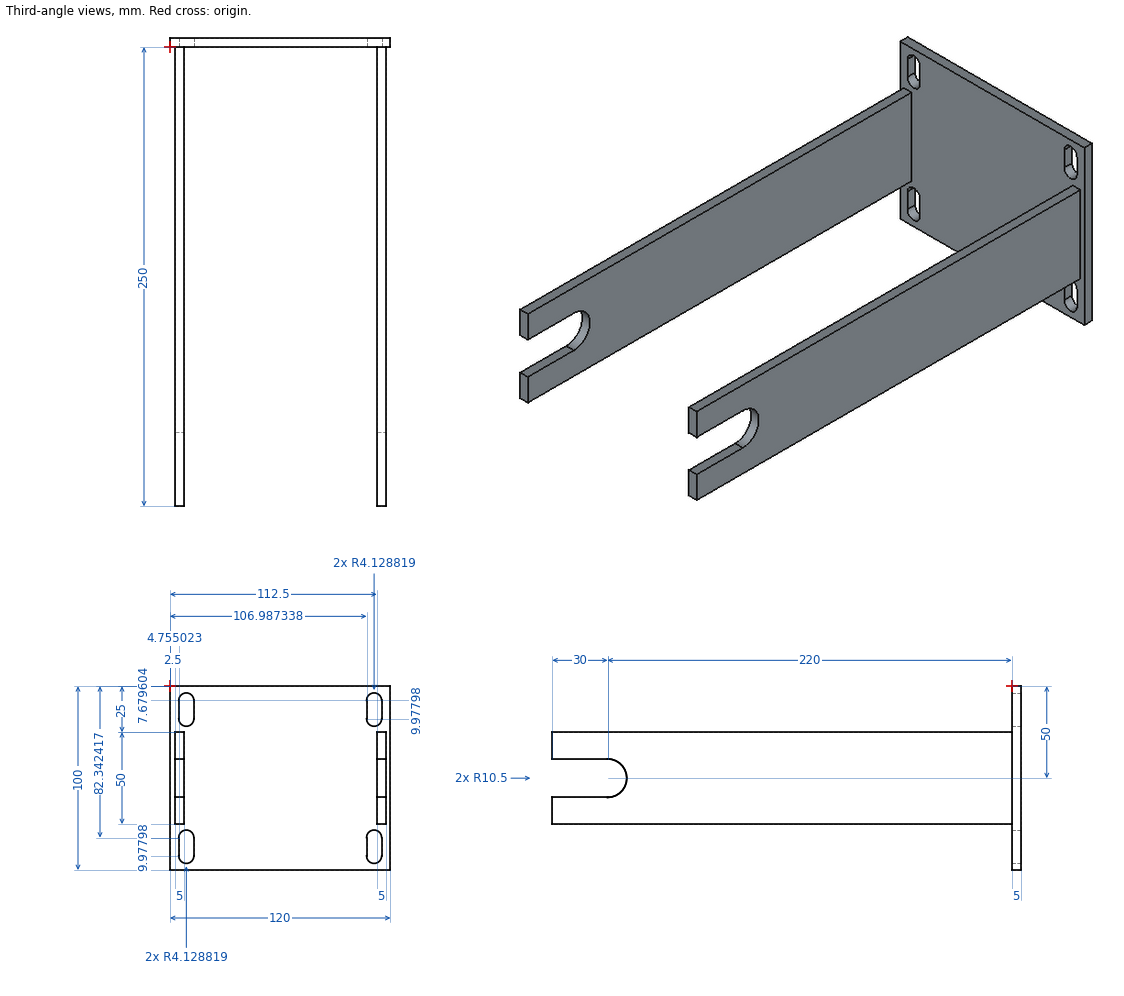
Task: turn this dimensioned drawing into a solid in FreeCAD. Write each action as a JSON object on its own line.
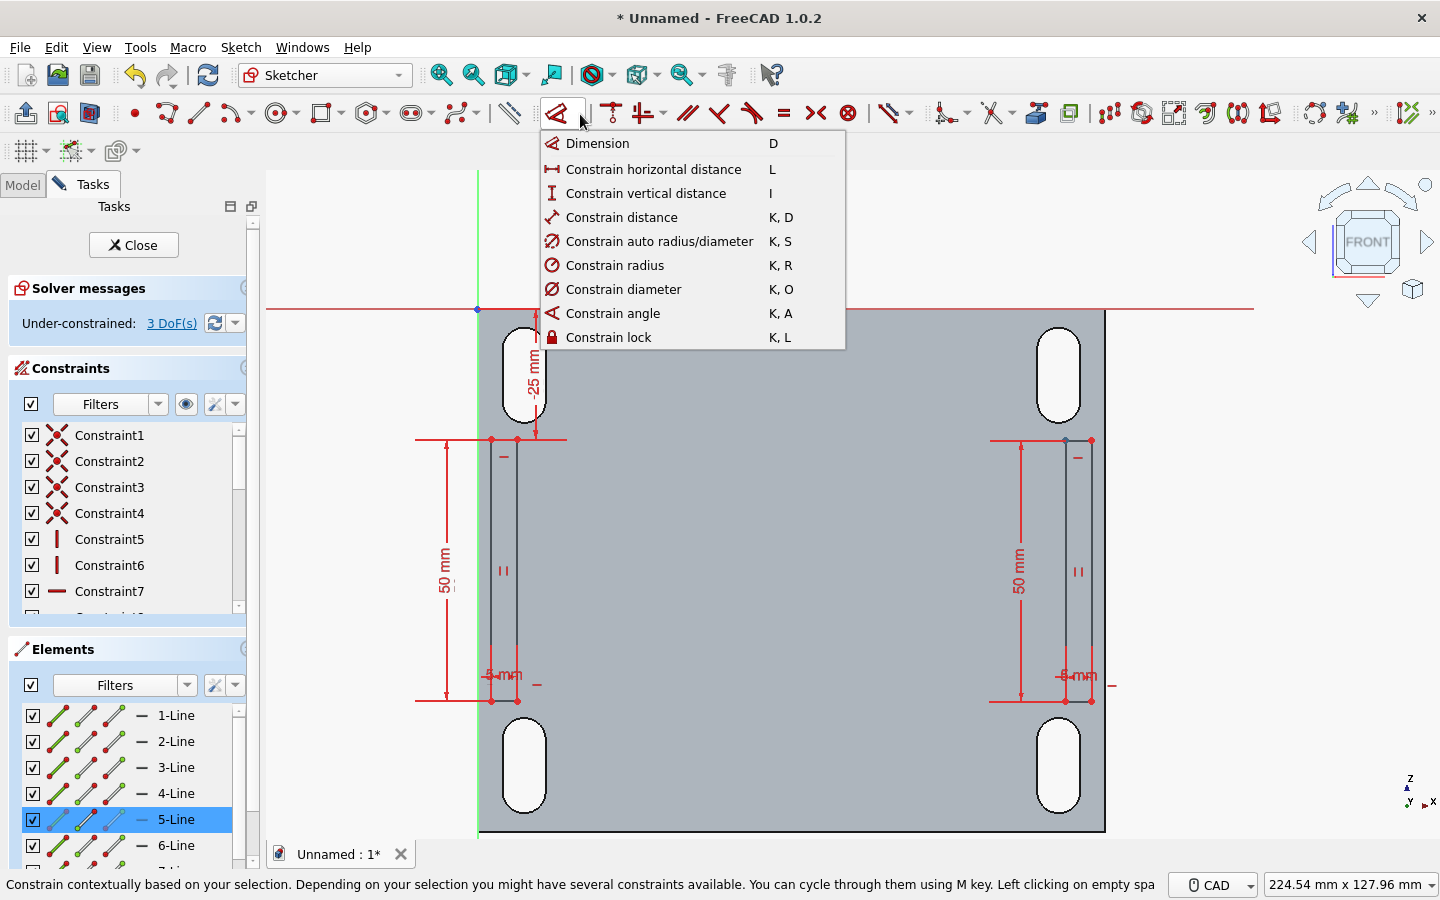
{"action": "left_click", "coordinate": [693, 193]}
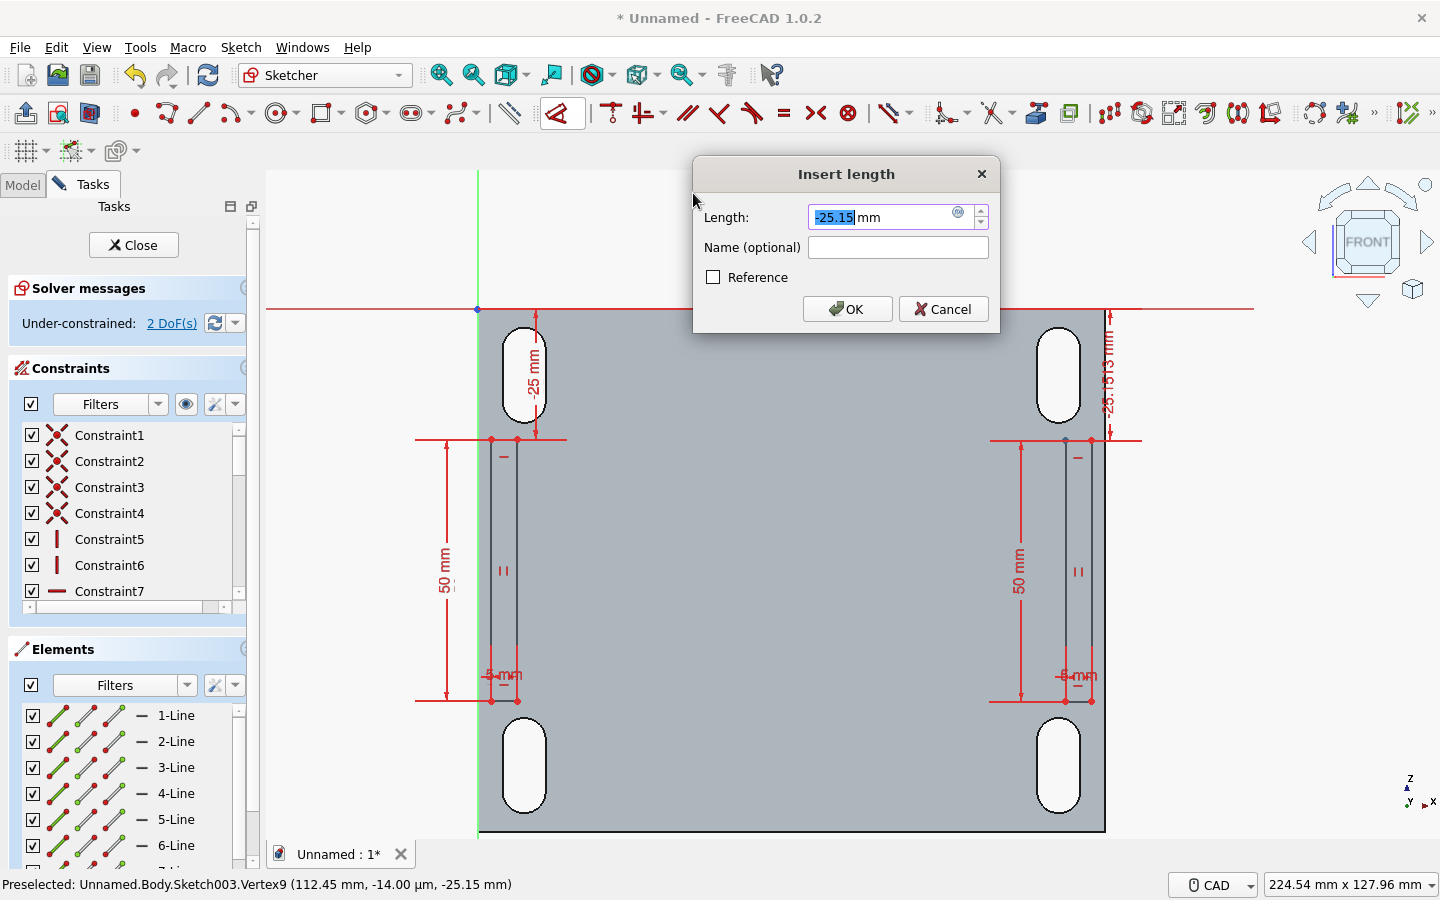
{"action": "type", "text": "-25"}
{"action": "key", "text": "Return"}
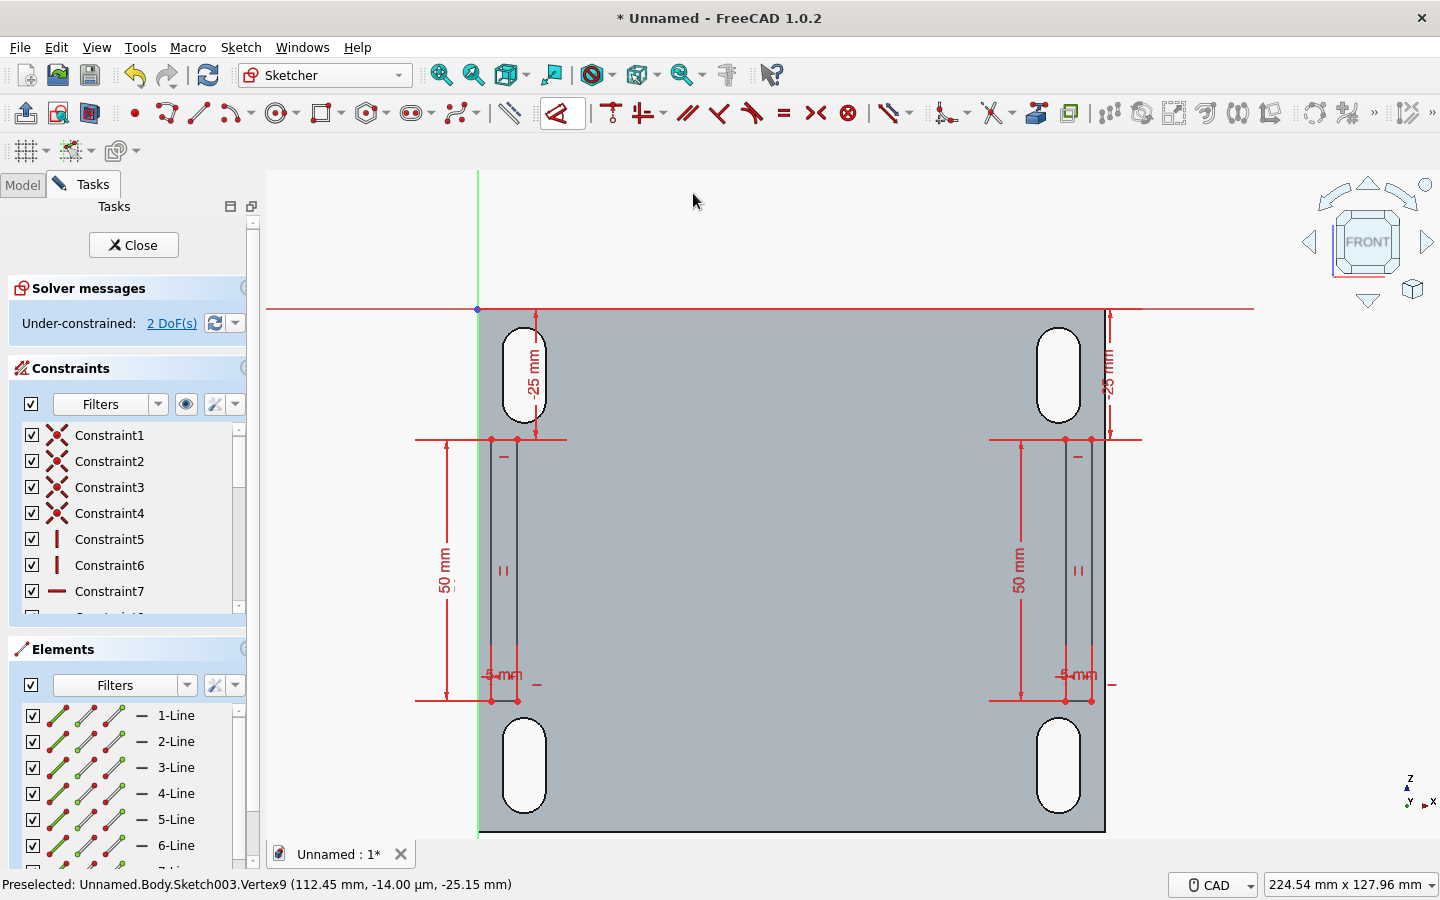
{"action": "scroll", "coordinate": [491, 440], "scroll_direction": "up", "scroll_amount": 6}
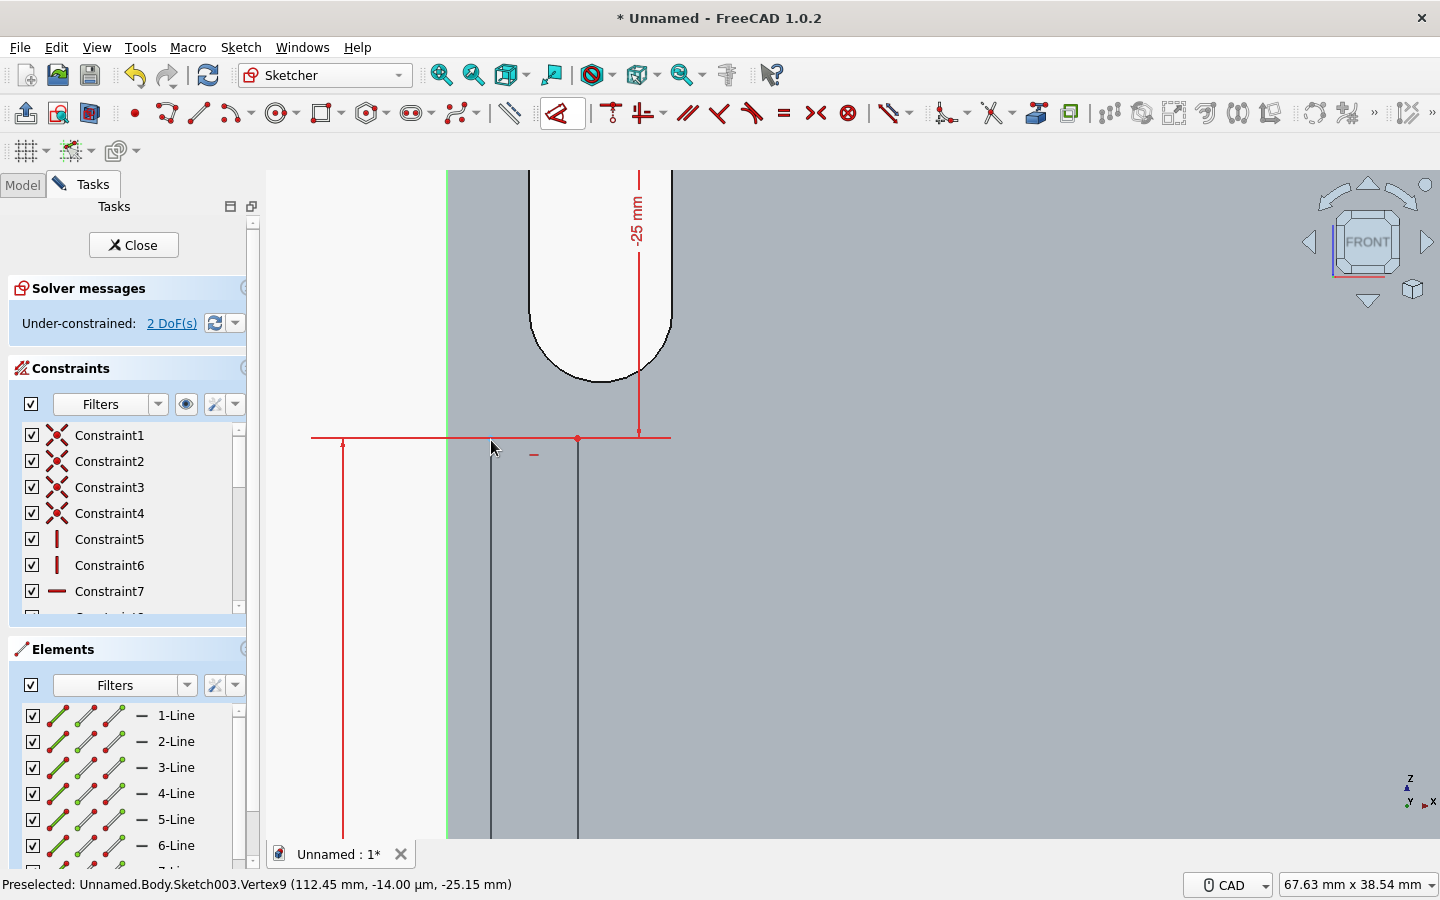
{"action": "left_click", "coordinate": [491, 438]}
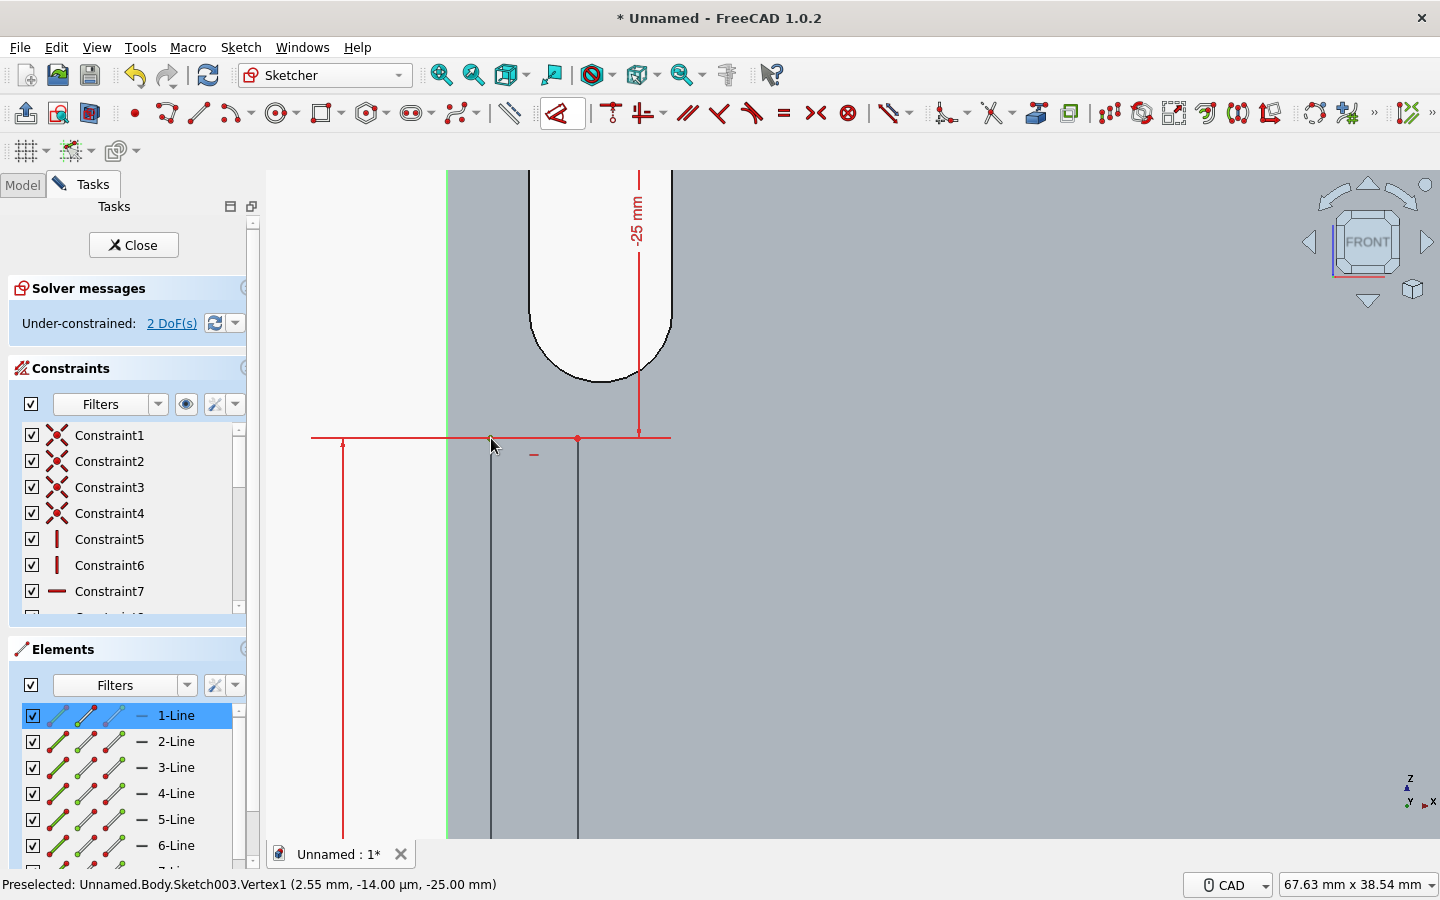
{"action": "key", "text": "l"}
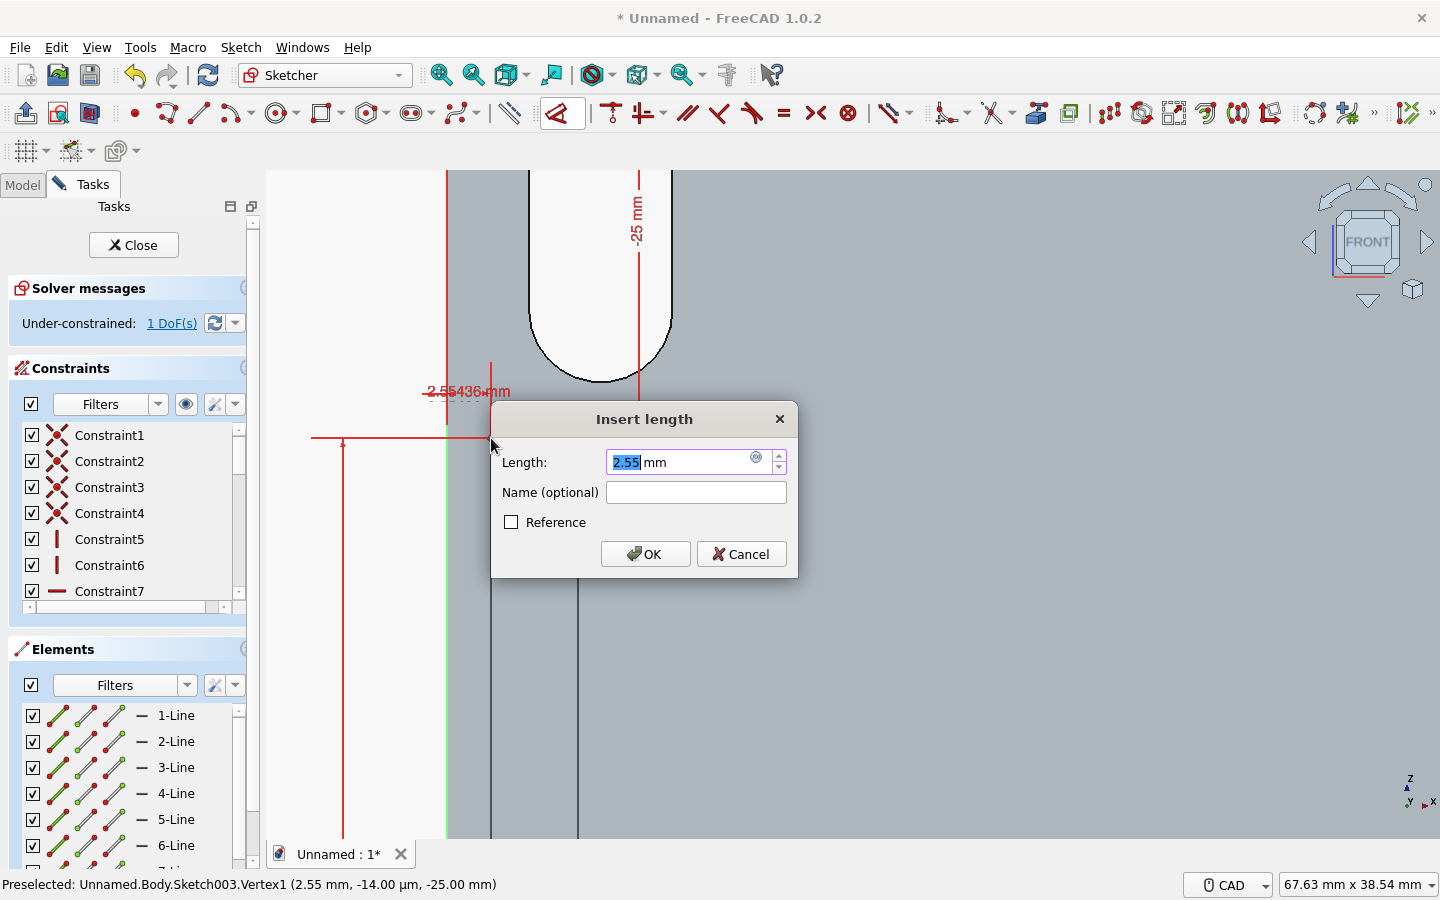
{"action": "type", "text": "2.5"}
{"action": "key", "text": "Return"}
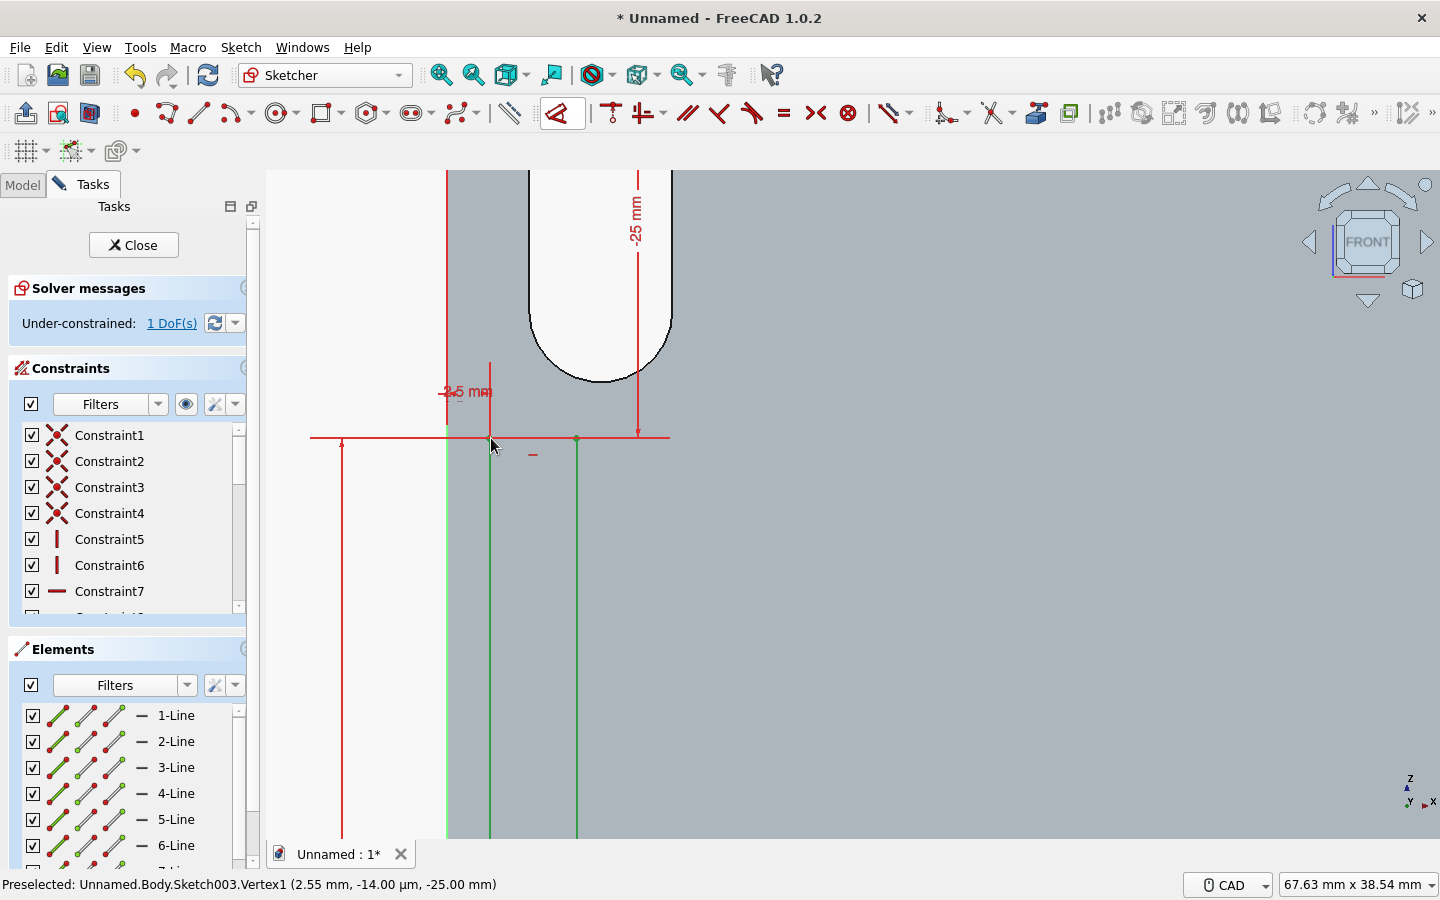
{"action": "scroll", "coordinate": [491, 440], "scroll_direction": "down", "scroll_amount": 6}